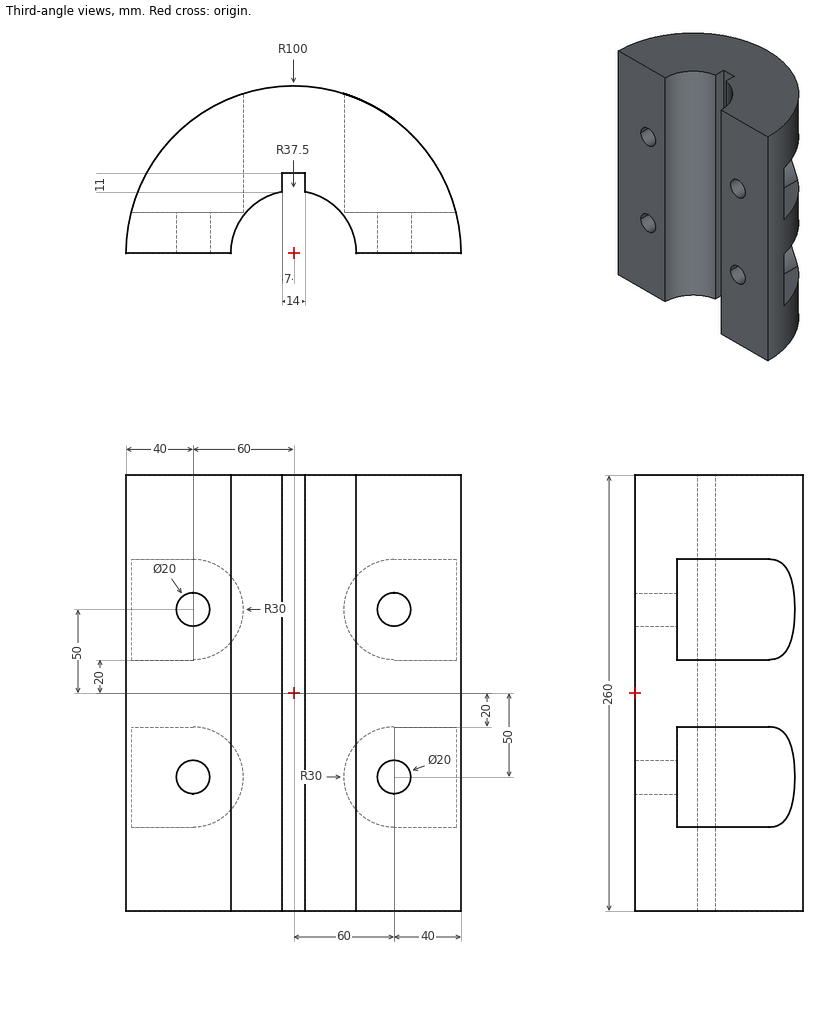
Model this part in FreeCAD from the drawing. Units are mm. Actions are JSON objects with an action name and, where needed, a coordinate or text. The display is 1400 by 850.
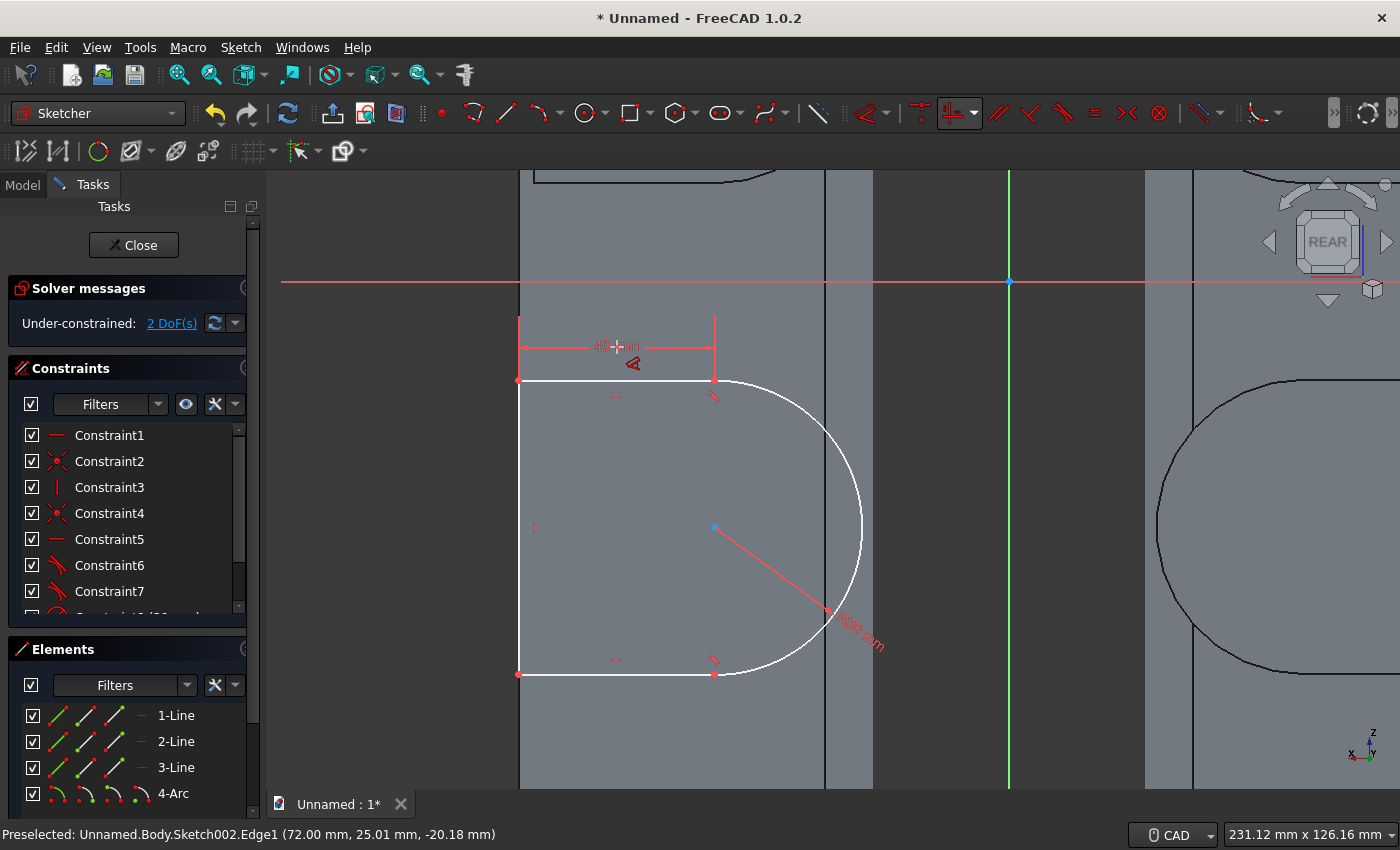
{"action": "left_click", "coordinate": [715, 381]}
{"action": "left_click", "coordinate": [862, 248]}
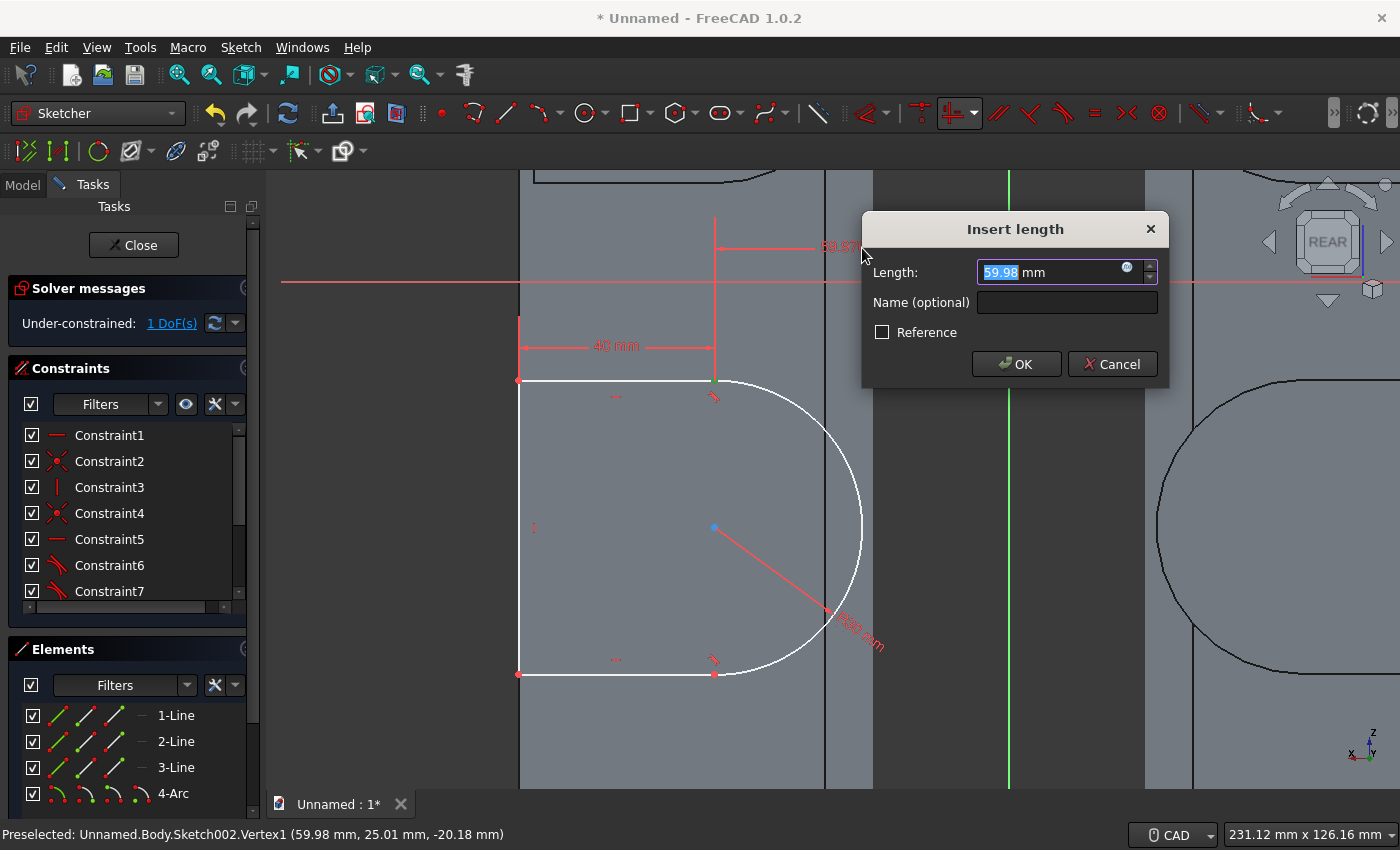
{"action": "type", "text": "60"}
{"action": "key", "text": "Return"}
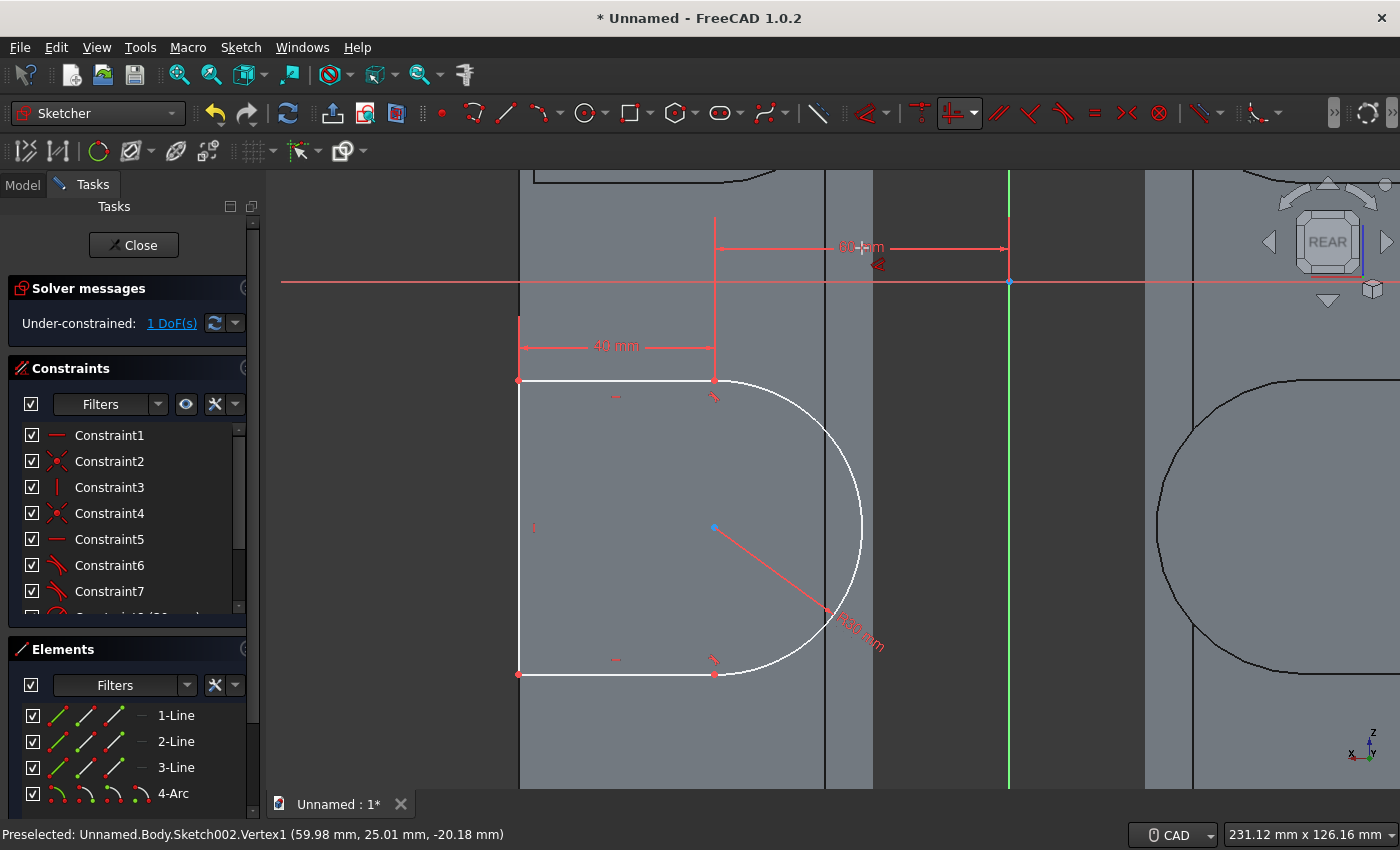
{"action": "left_click", "coordinate": [715, 381]}
{"action": "left_click", "coordinate": [1043, 331]}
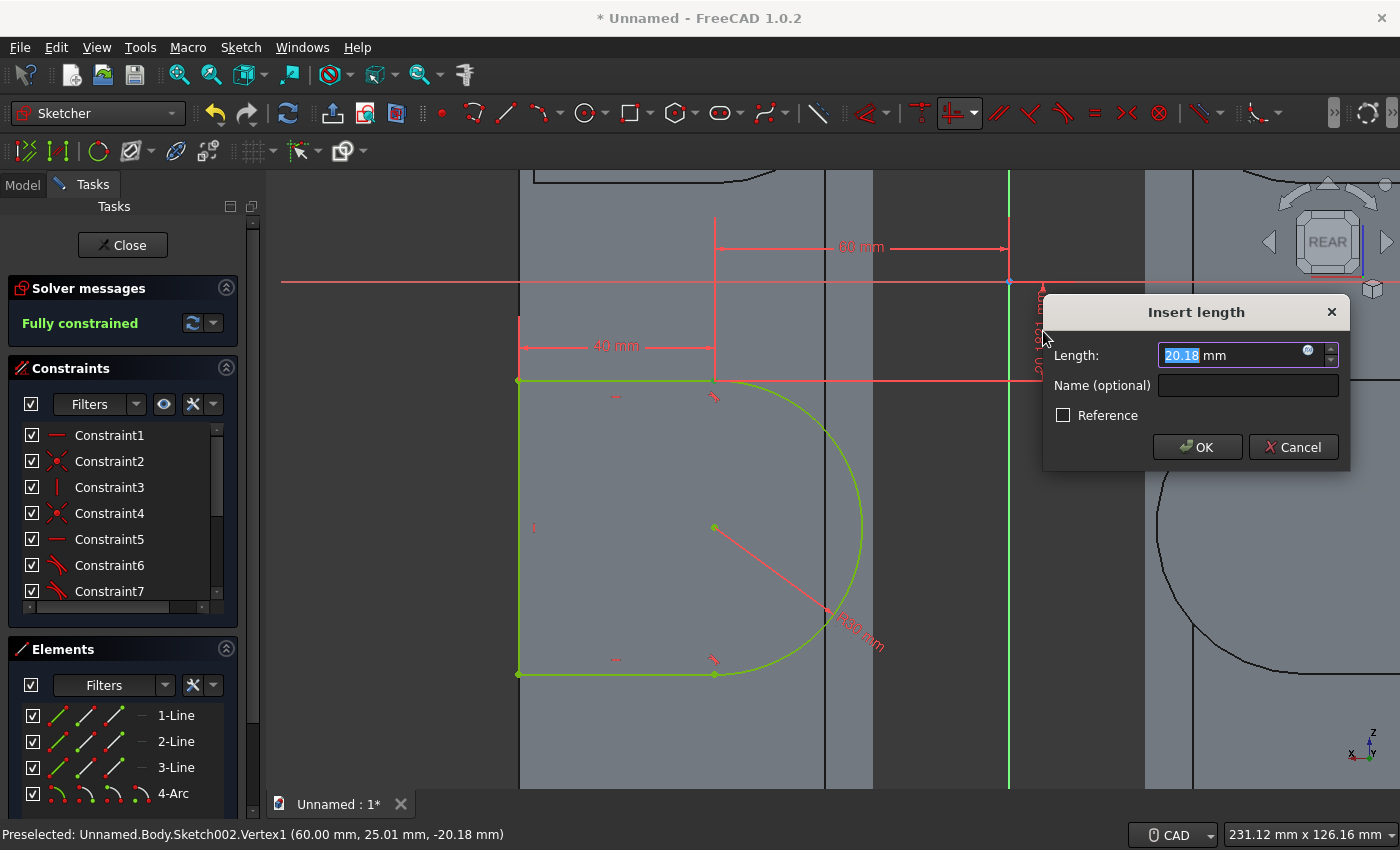
{"action": "type", "text": "20"}
{"action": "key", "text": "Return"}
{"action": "key", "text": "Escape"}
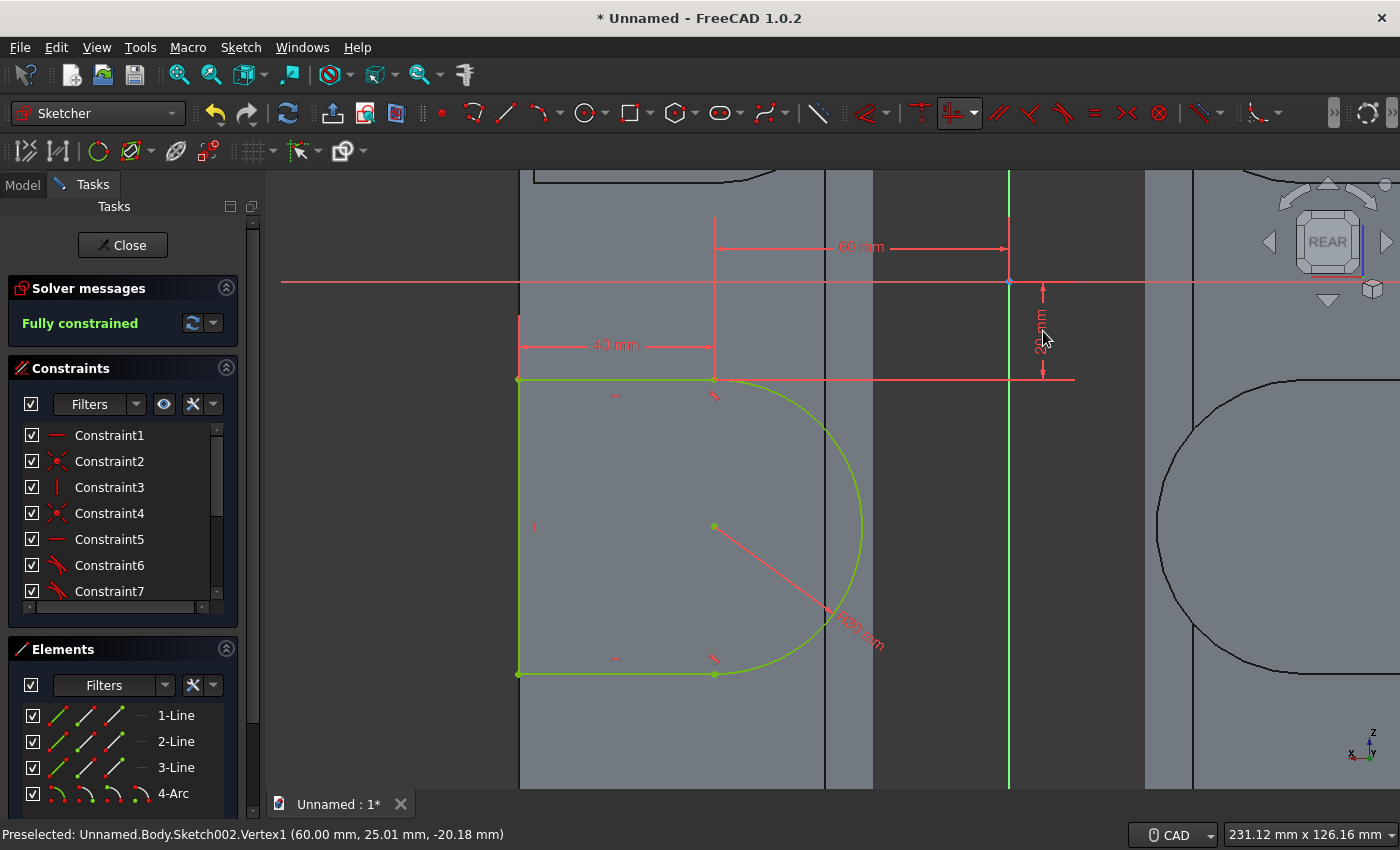
{"action": "left_click", "coordinate": [123, 245]}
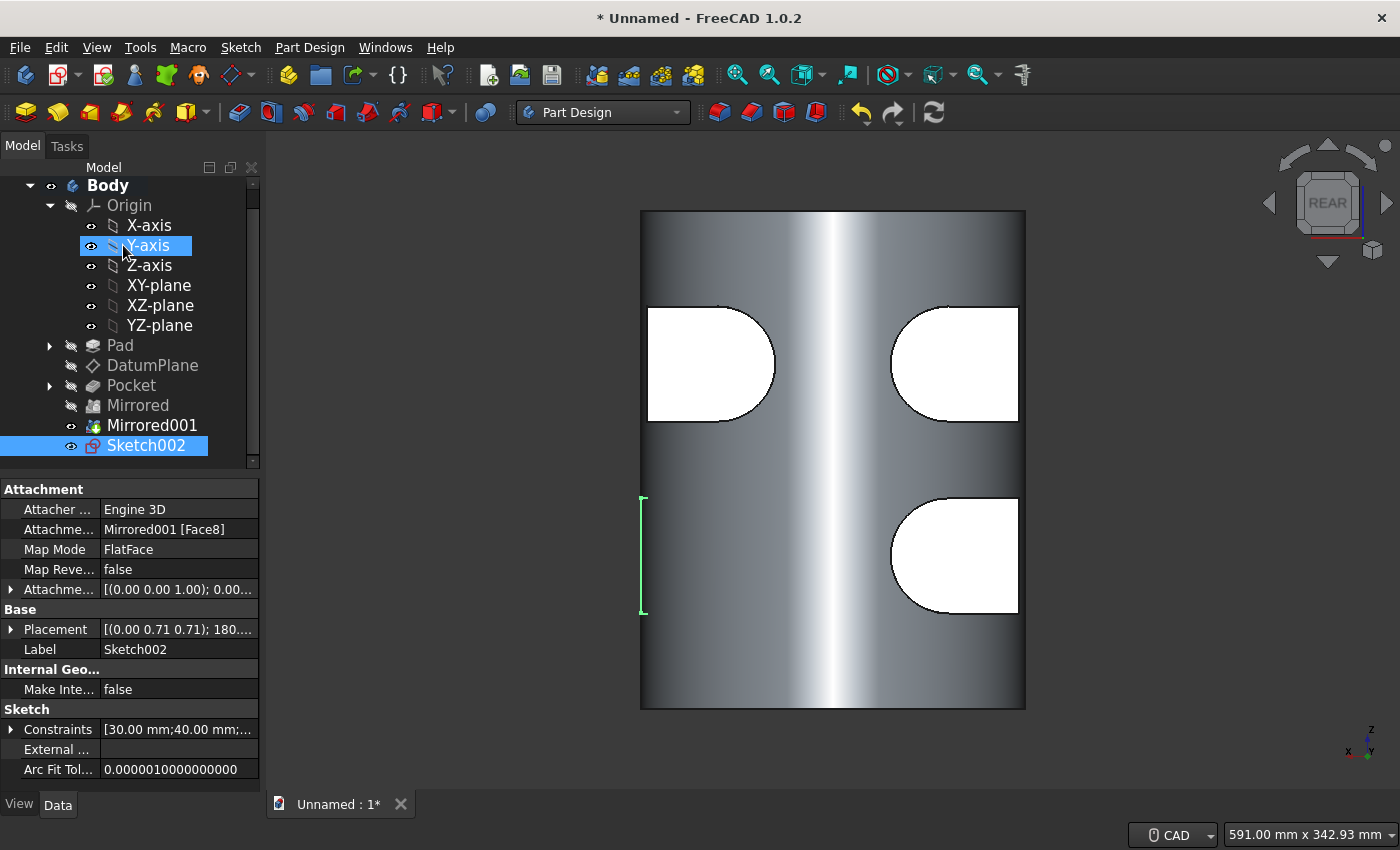
{"action": "left_click", "coordinate": [240, 112]}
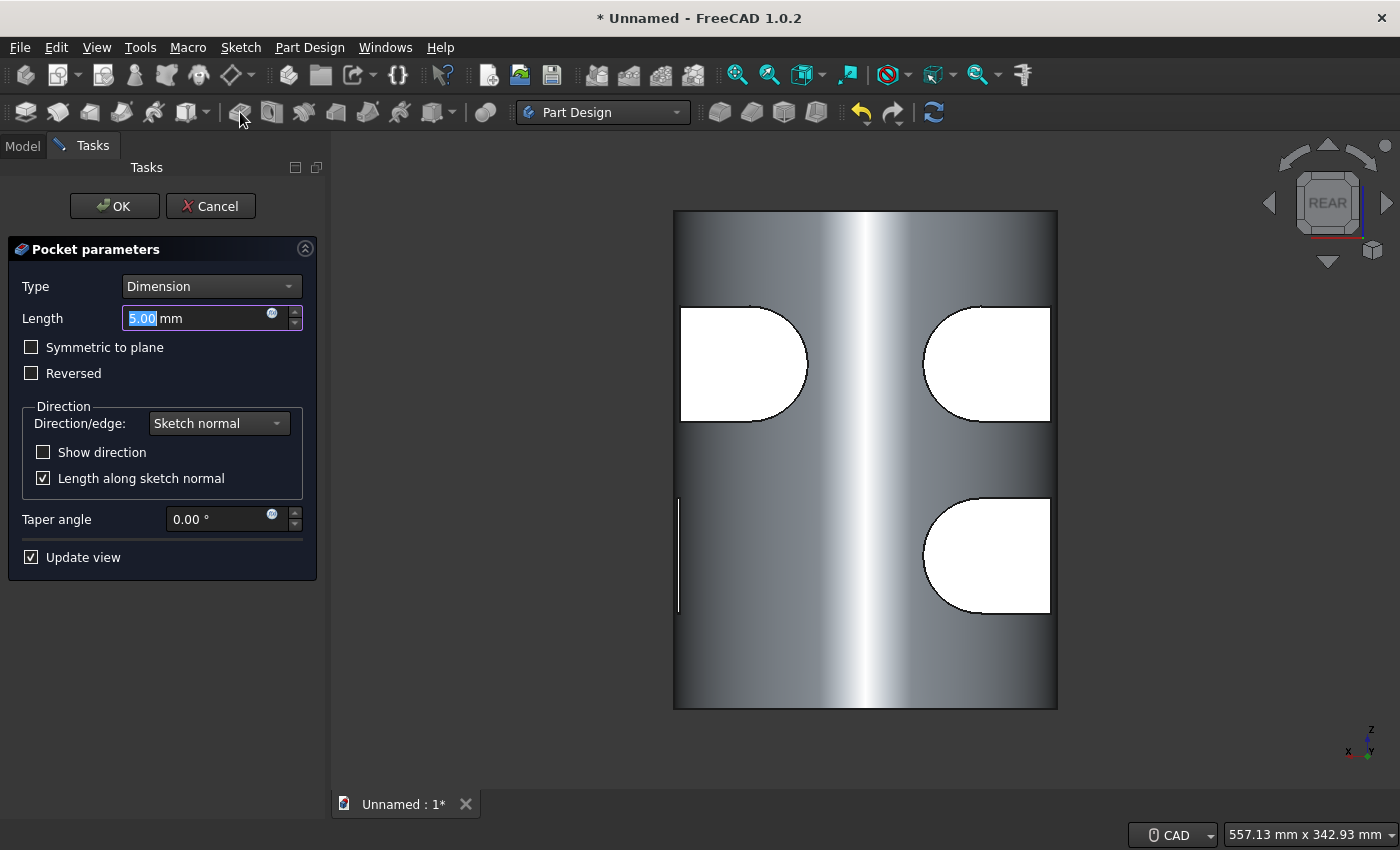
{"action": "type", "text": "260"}
{"action": "key", "text": "Tab"}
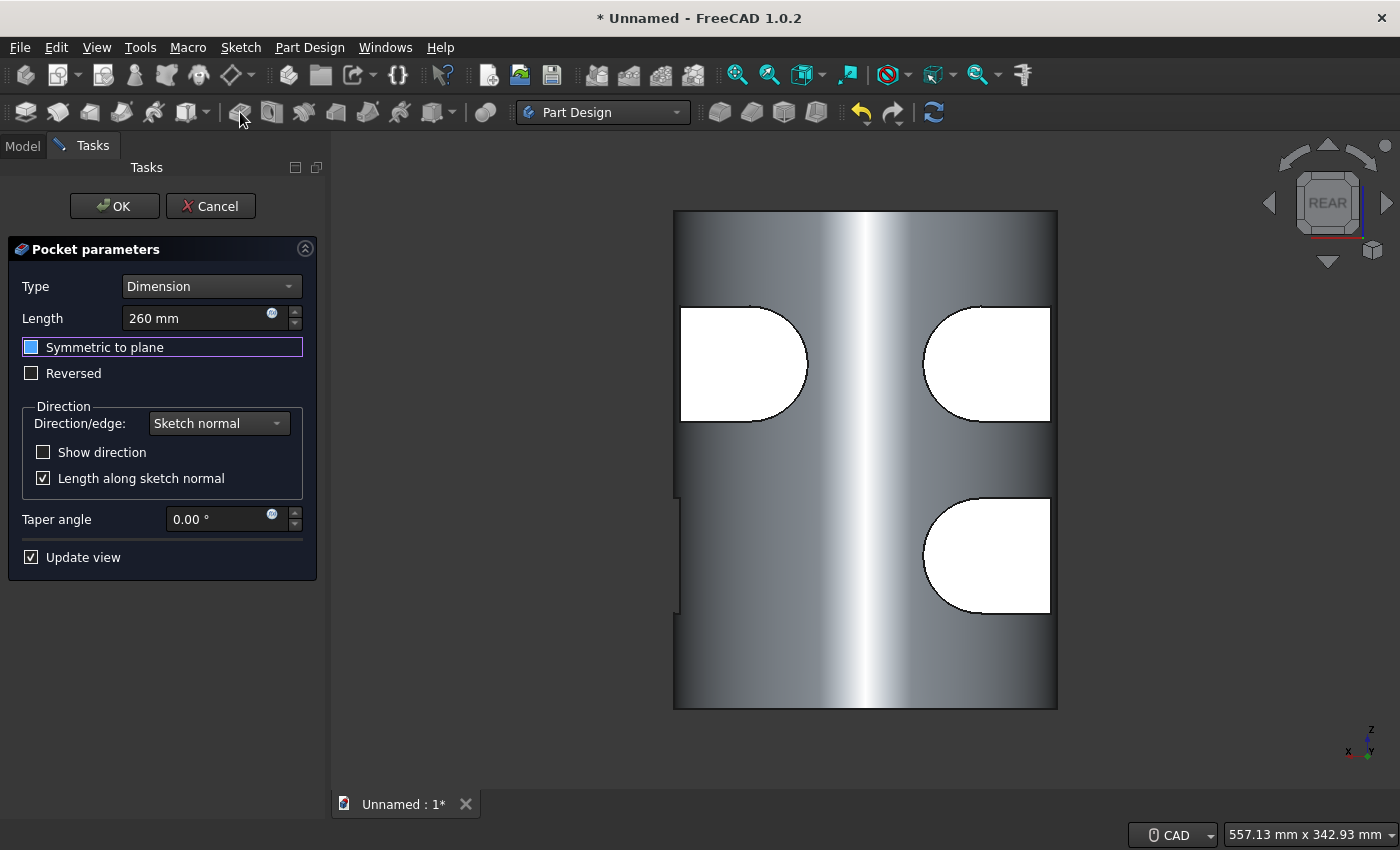
{"action": "left_click", "coordinate": [30, 373]}